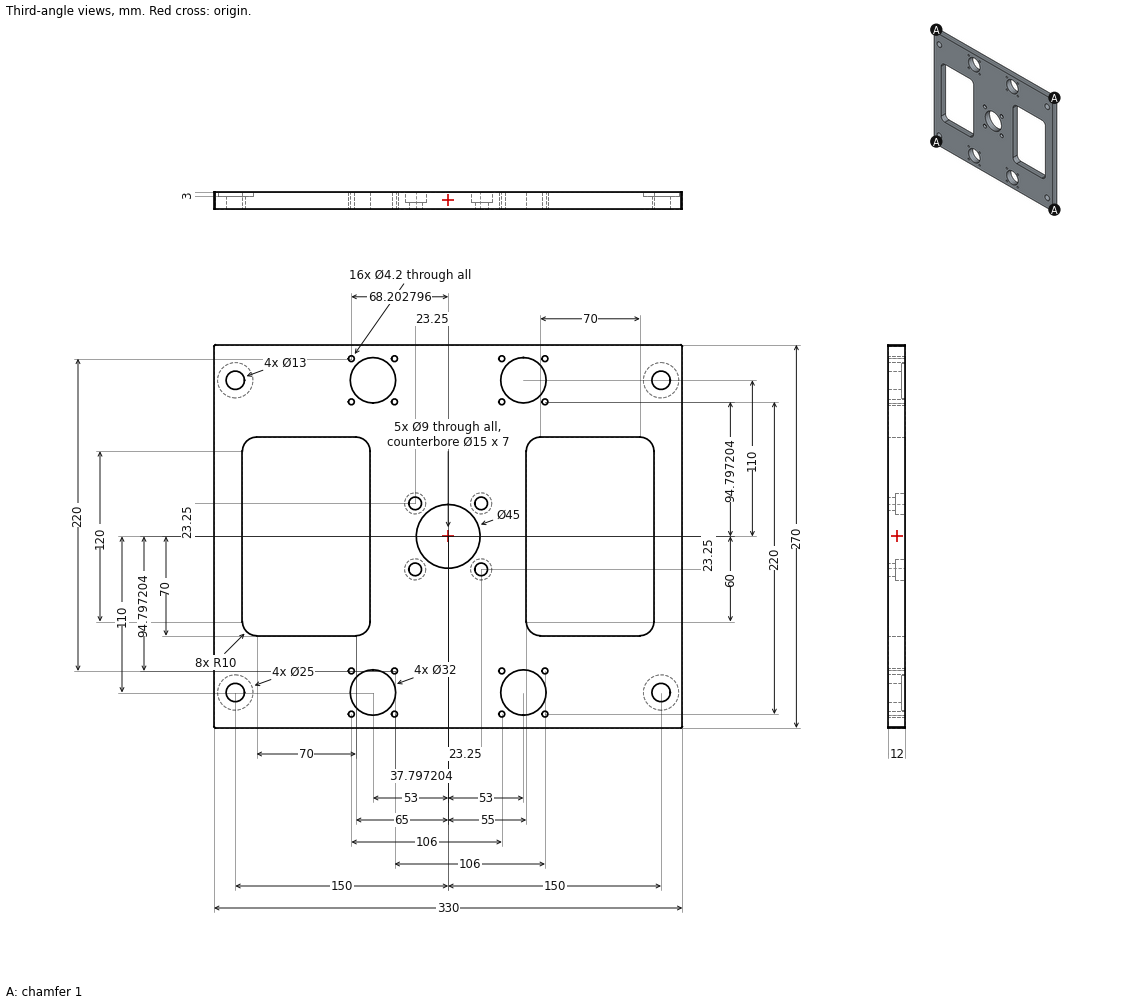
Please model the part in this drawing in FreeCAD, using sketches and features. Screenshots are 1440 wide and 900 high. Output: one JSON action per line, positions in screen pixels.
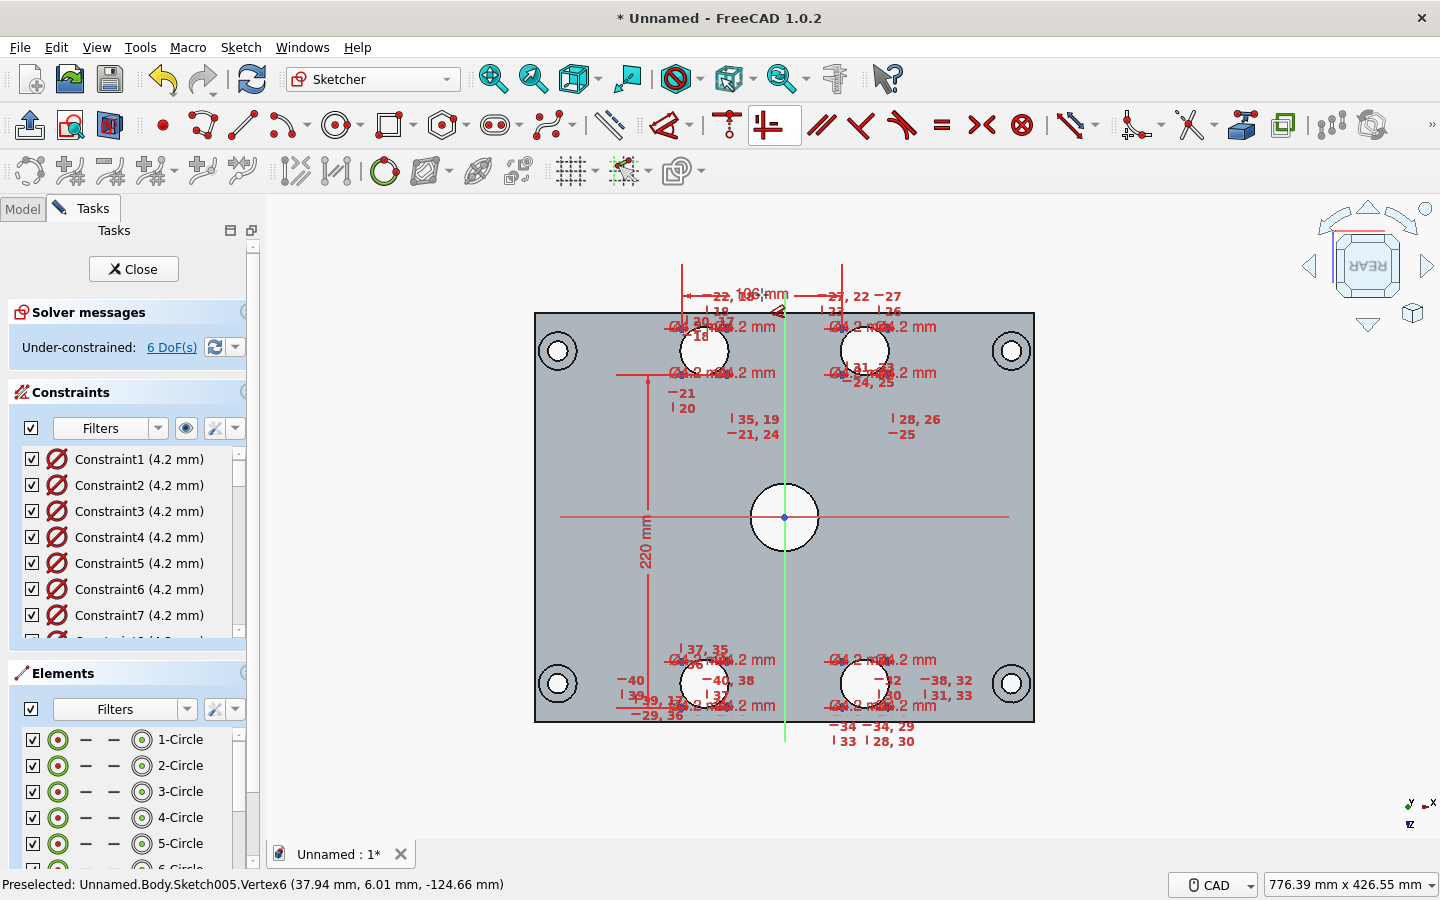
{"action": "left_click", "coordinate": [727, 375]}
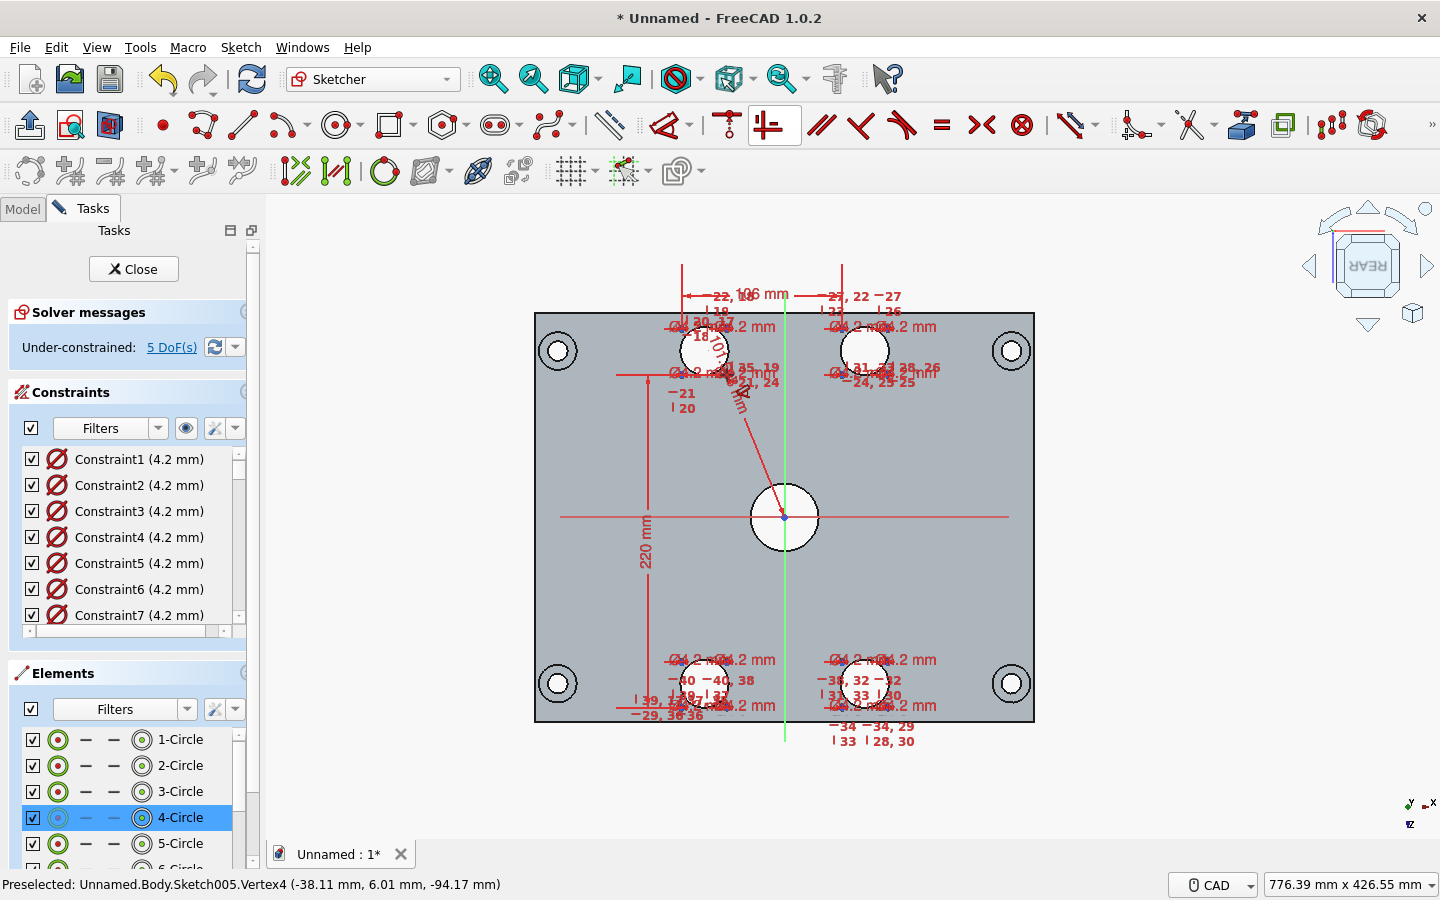
{"action": "left_click", "coordinate": [888, 375]}
{"action": "left_click", "coordinate": [808, 341]}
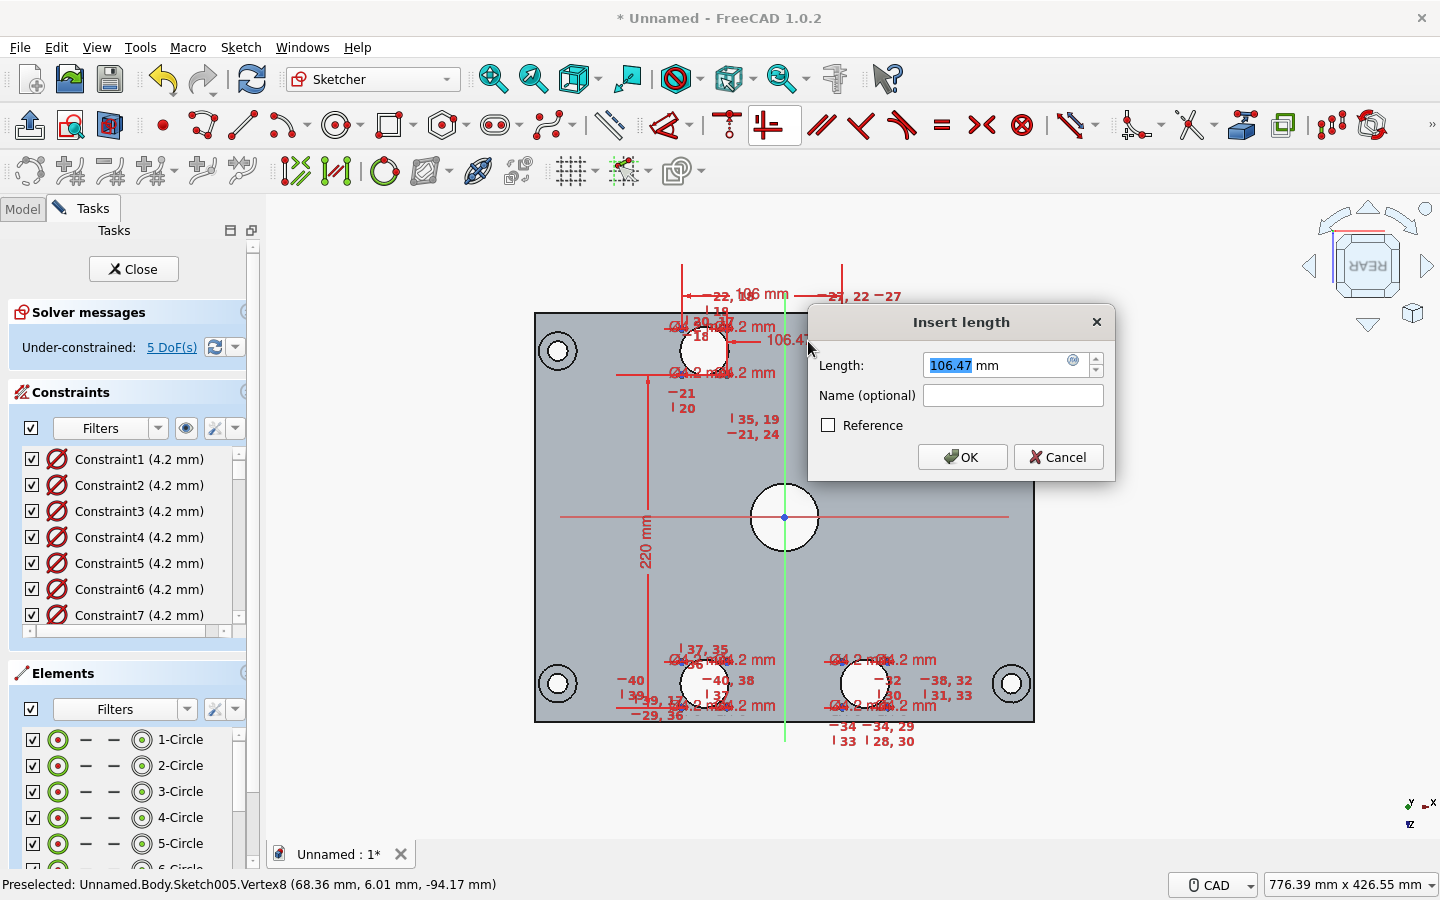
{"action": "type", "text": "106"}
{"action": "key", "text": "Return"}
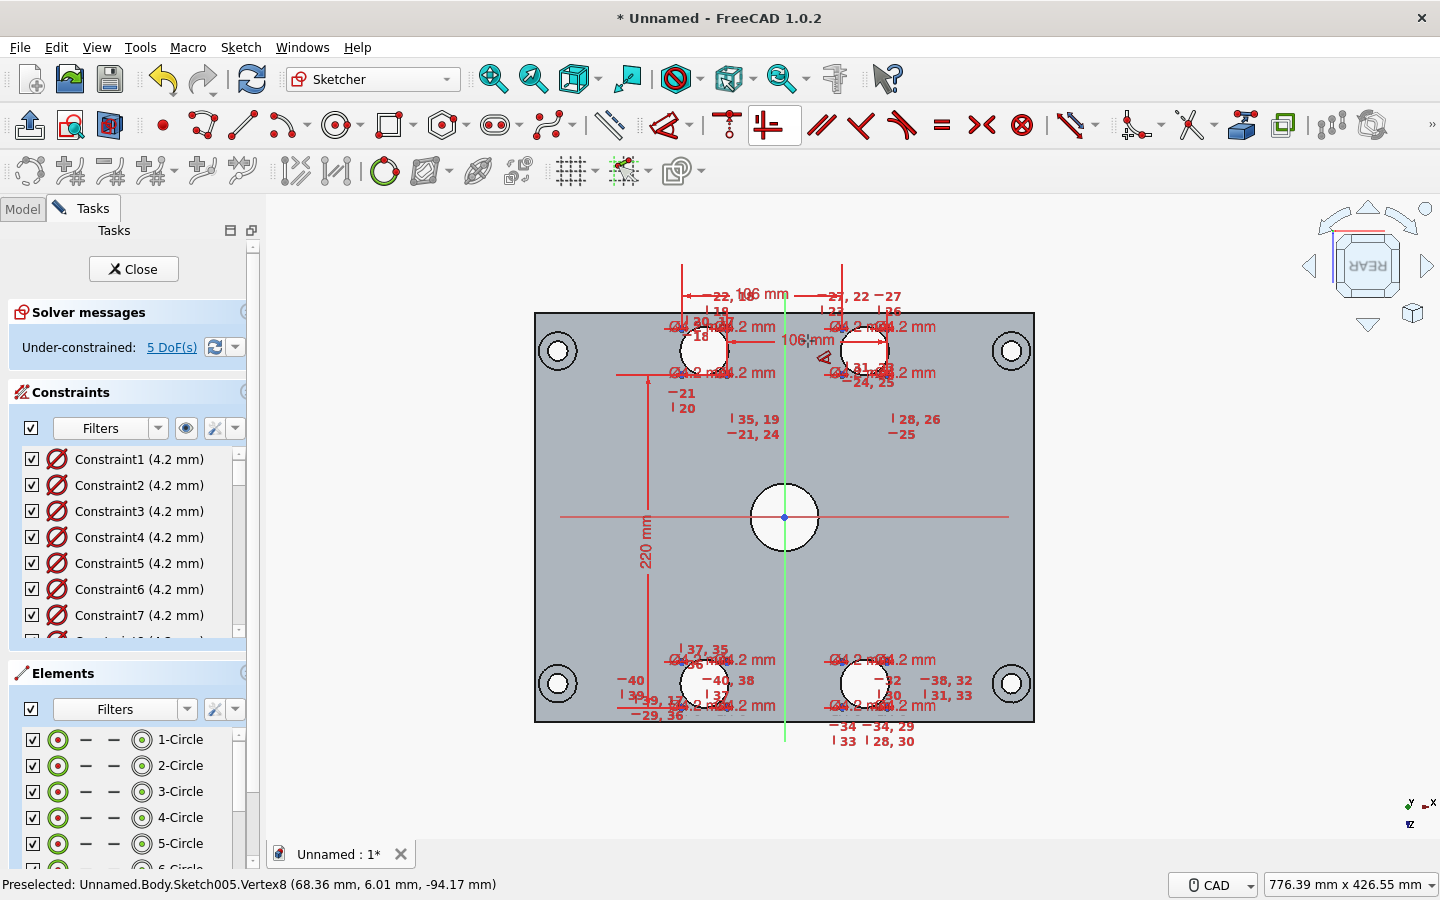
{"action": "left_click", "coordinate": [887, 329]}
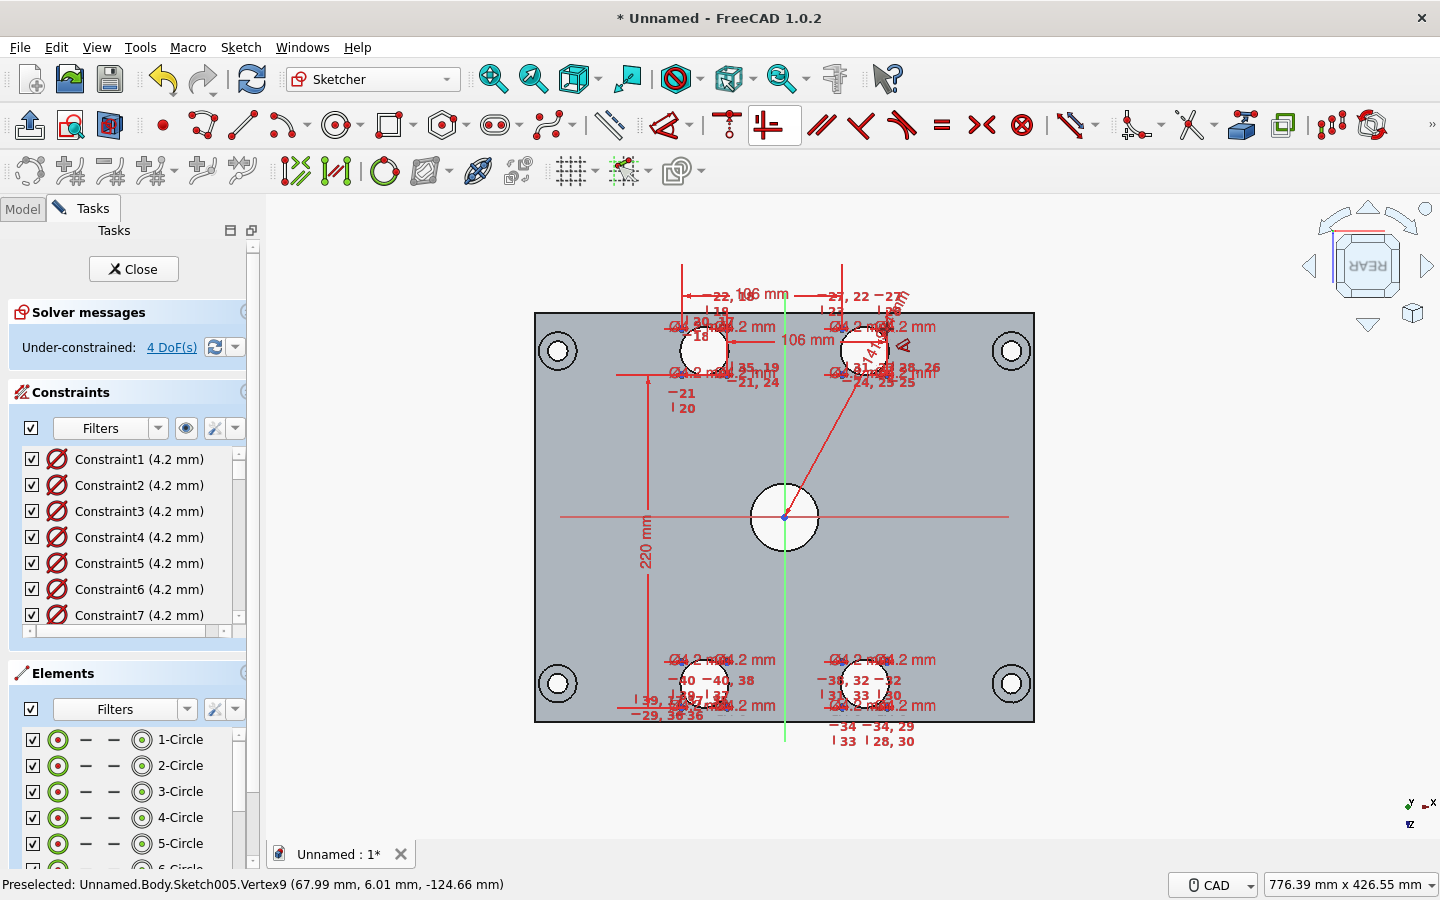
{"action": "left_click", "coordinate": [887, 662]}
{"action": "left_click", "coordinate": [921, 495]}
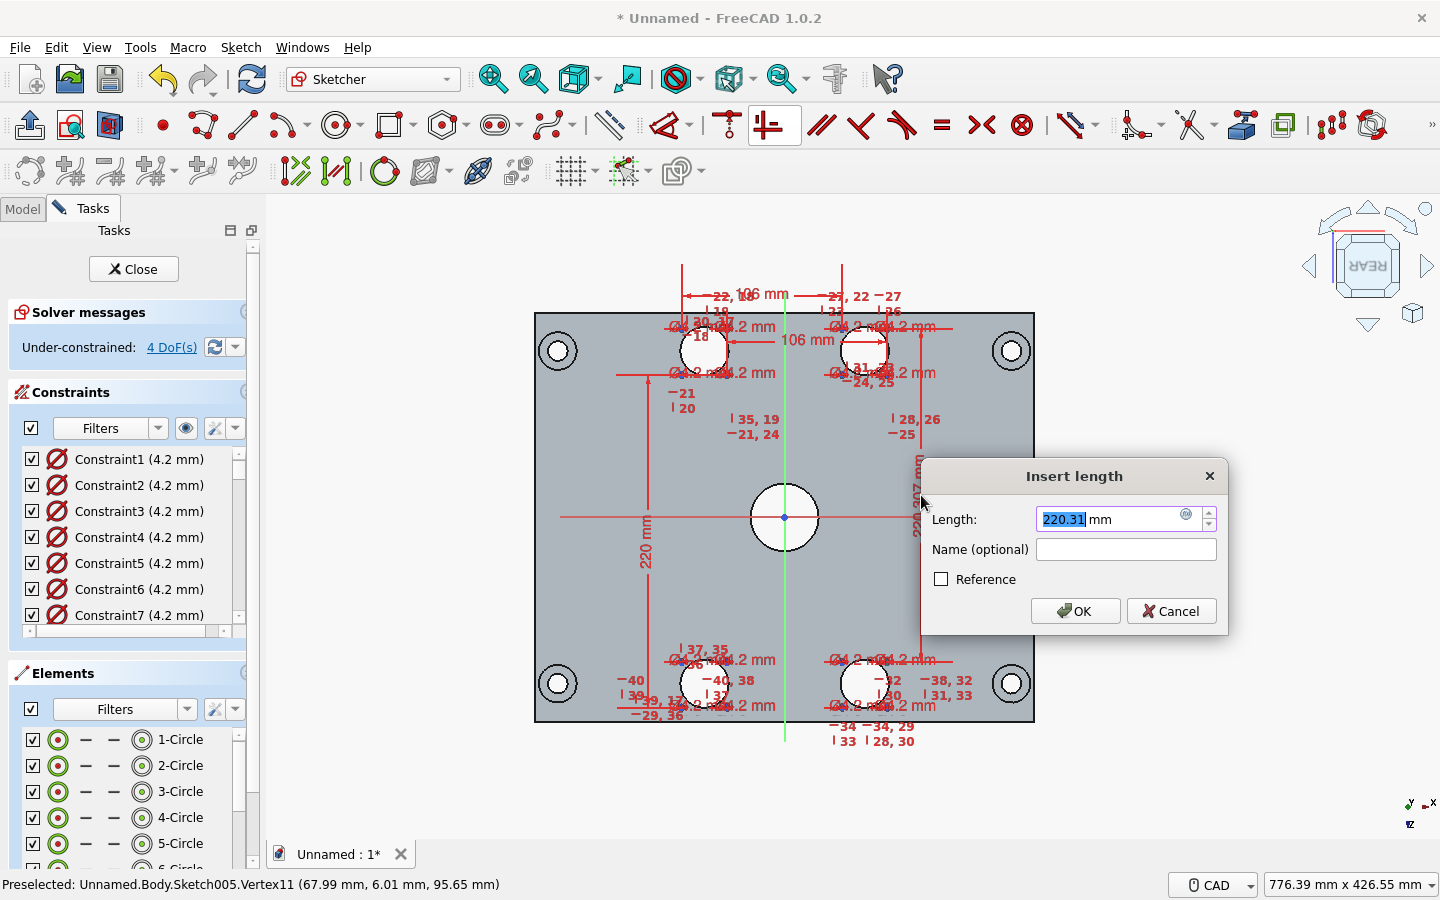
{"action": "type", "text": "220"}
{"action": "key", "text": "Return"}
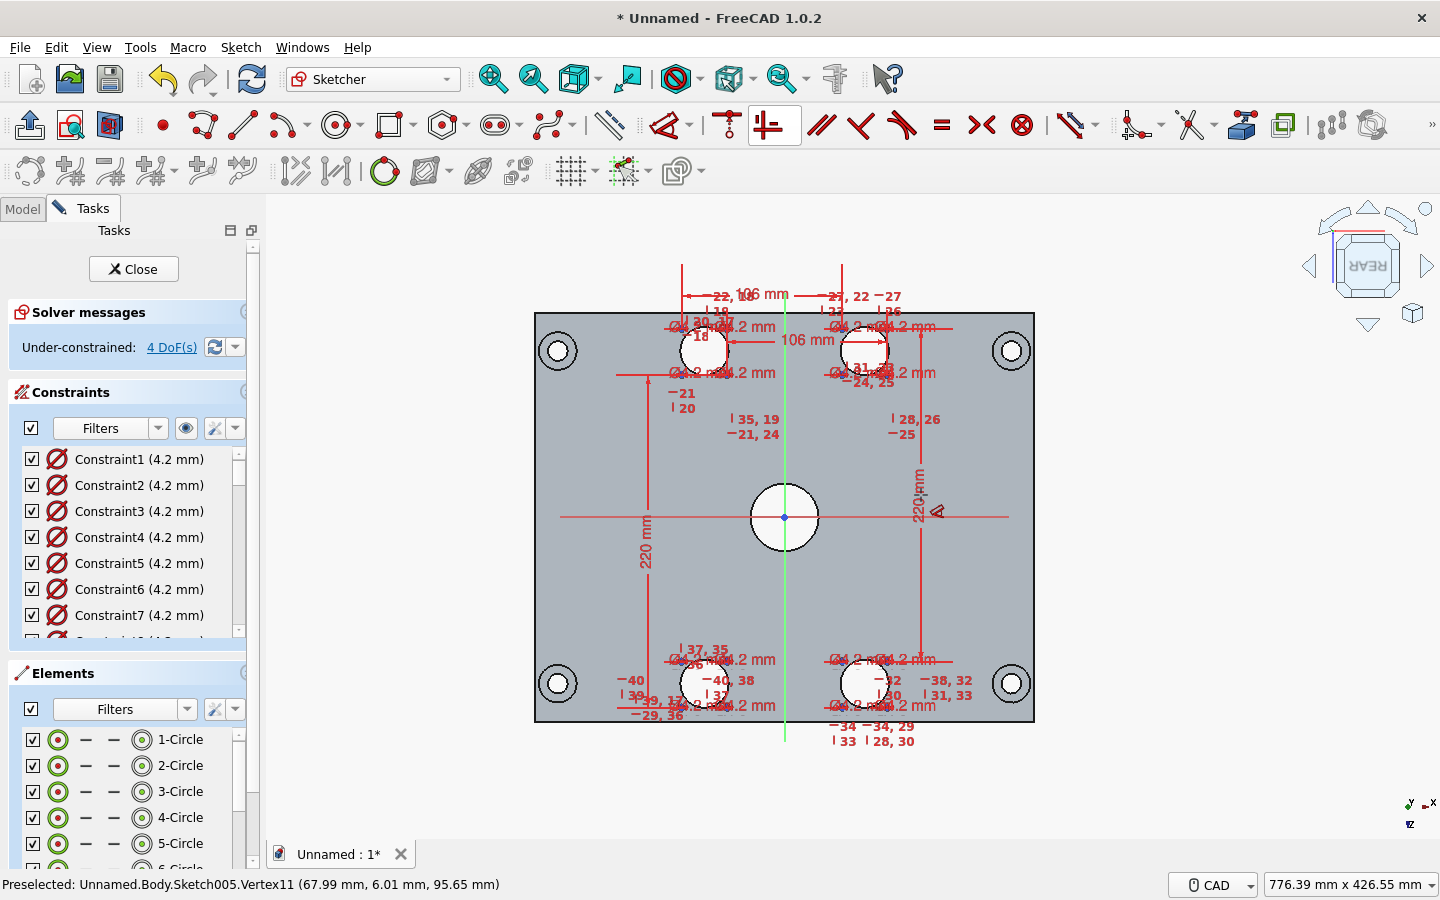
{"action": "left_click", "coordinate": [682, 708]}
{"action": "left_click", "coordinate": [733, 742]}